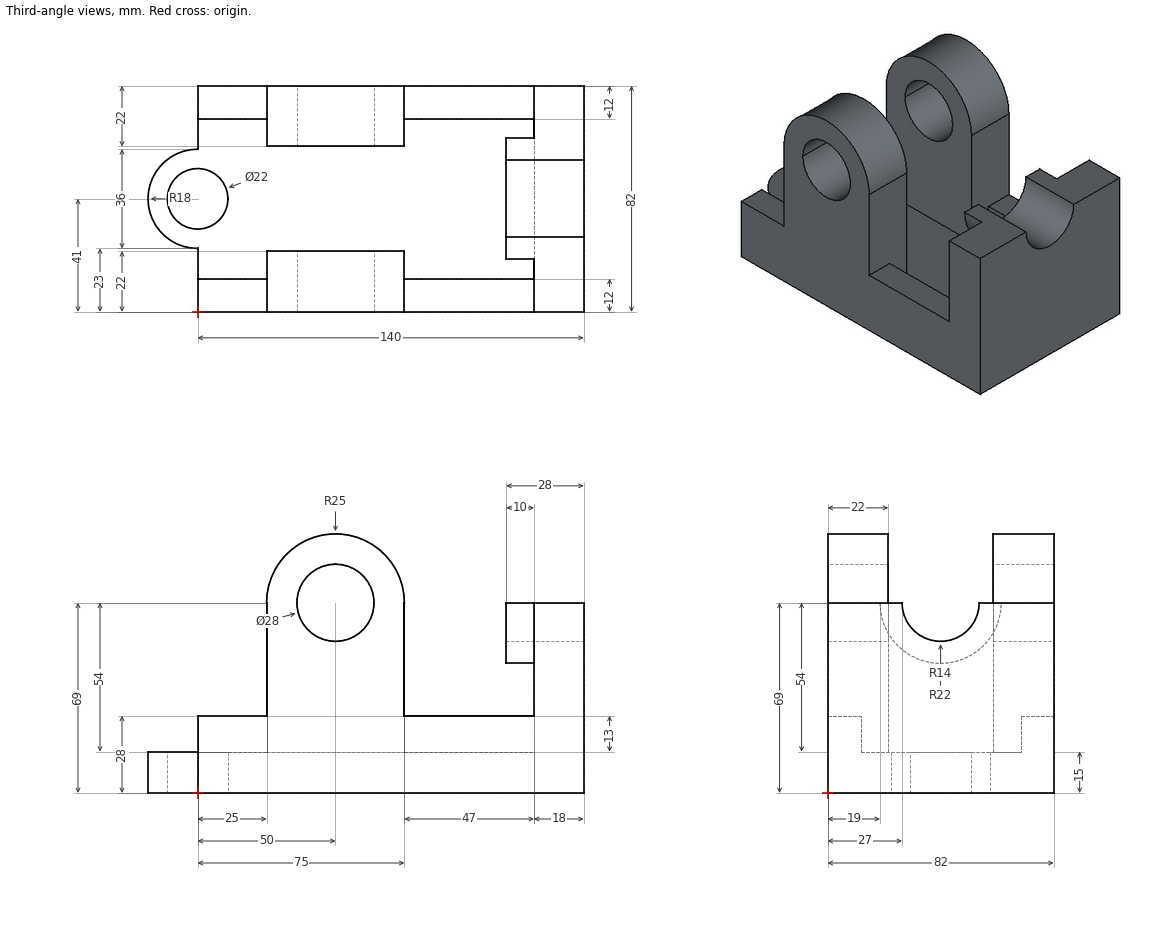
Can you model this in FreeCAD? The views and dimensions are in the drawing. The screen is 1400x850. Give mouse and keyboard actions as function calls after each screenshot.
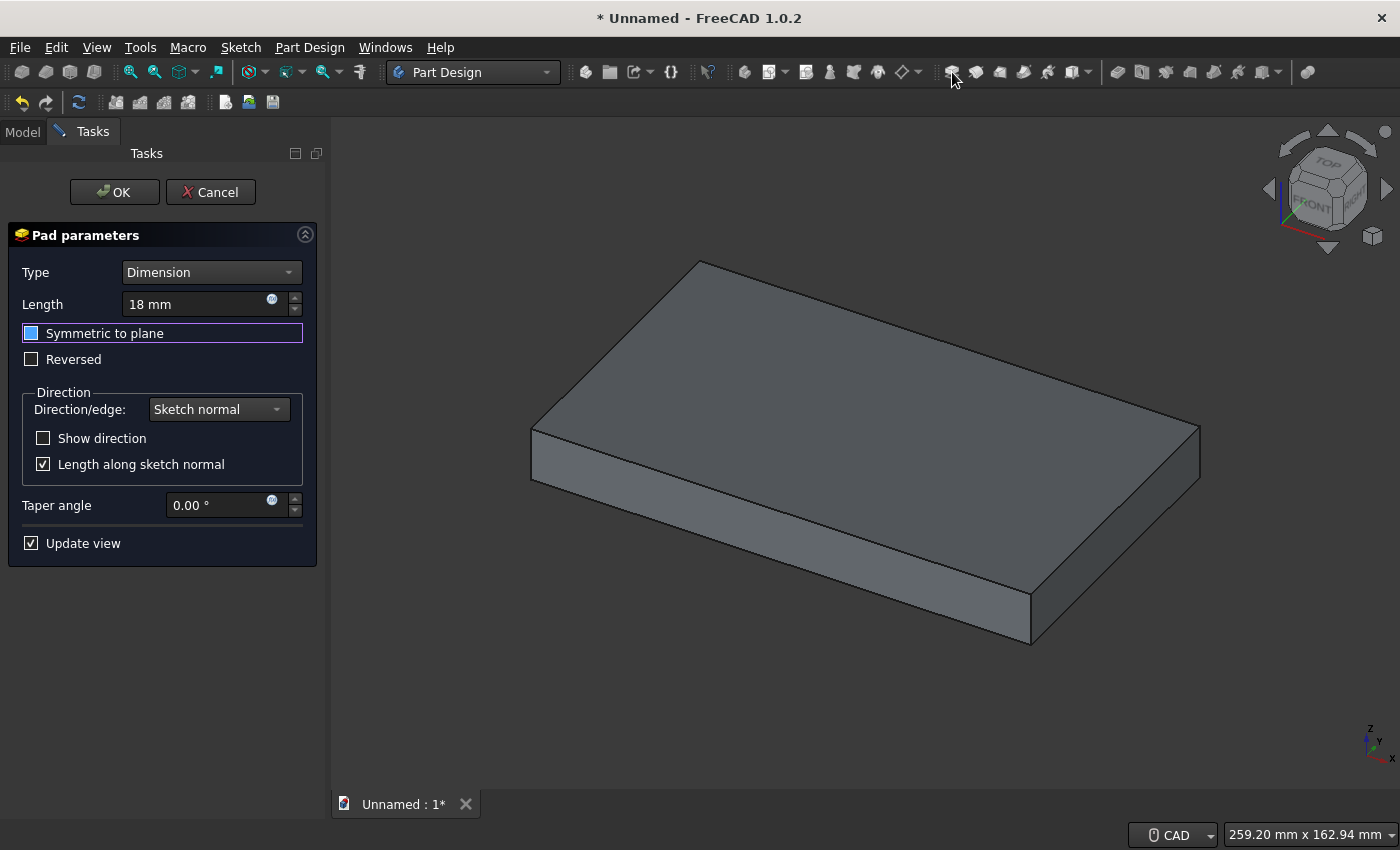
click(30, 359)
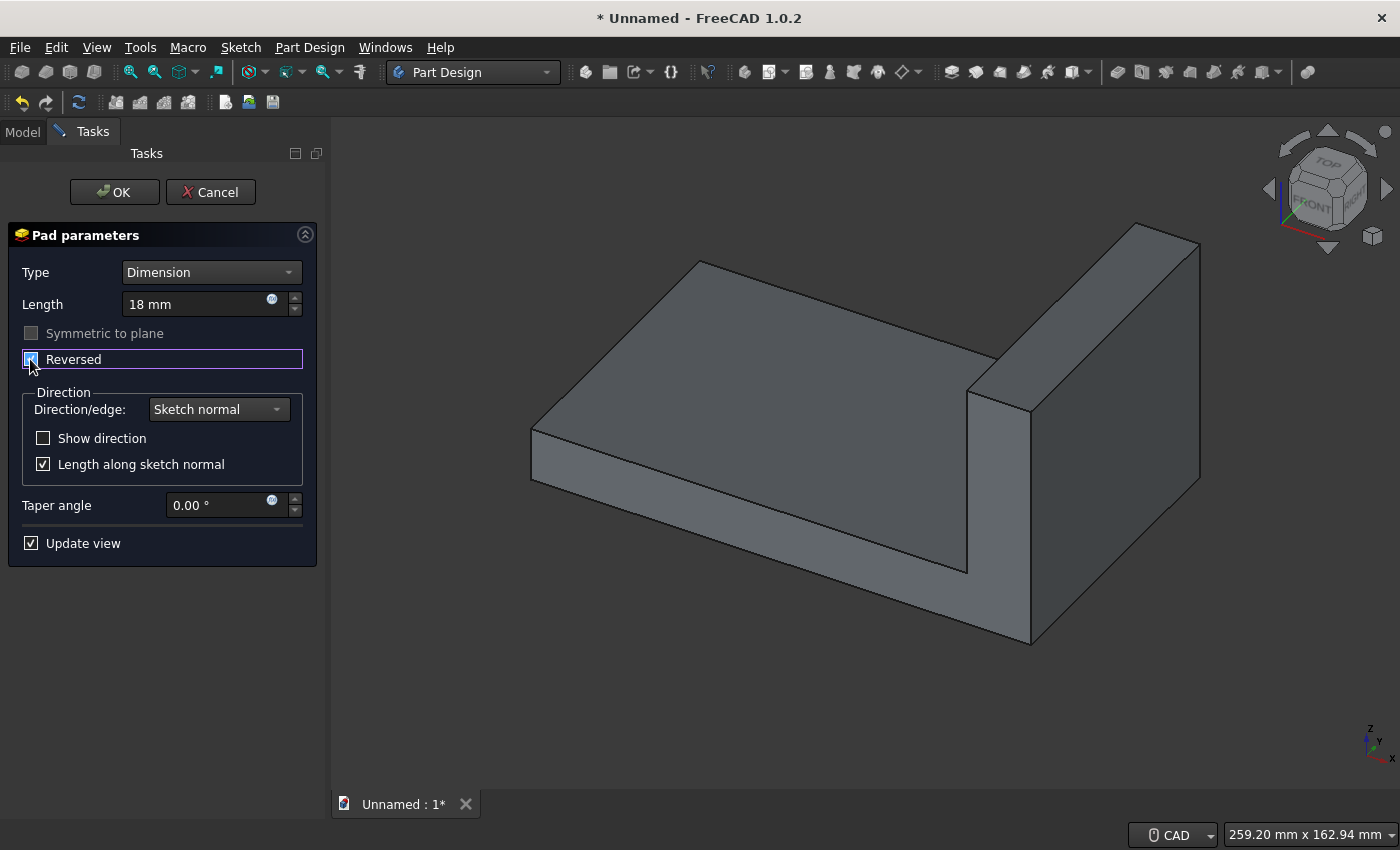
click(115, 192)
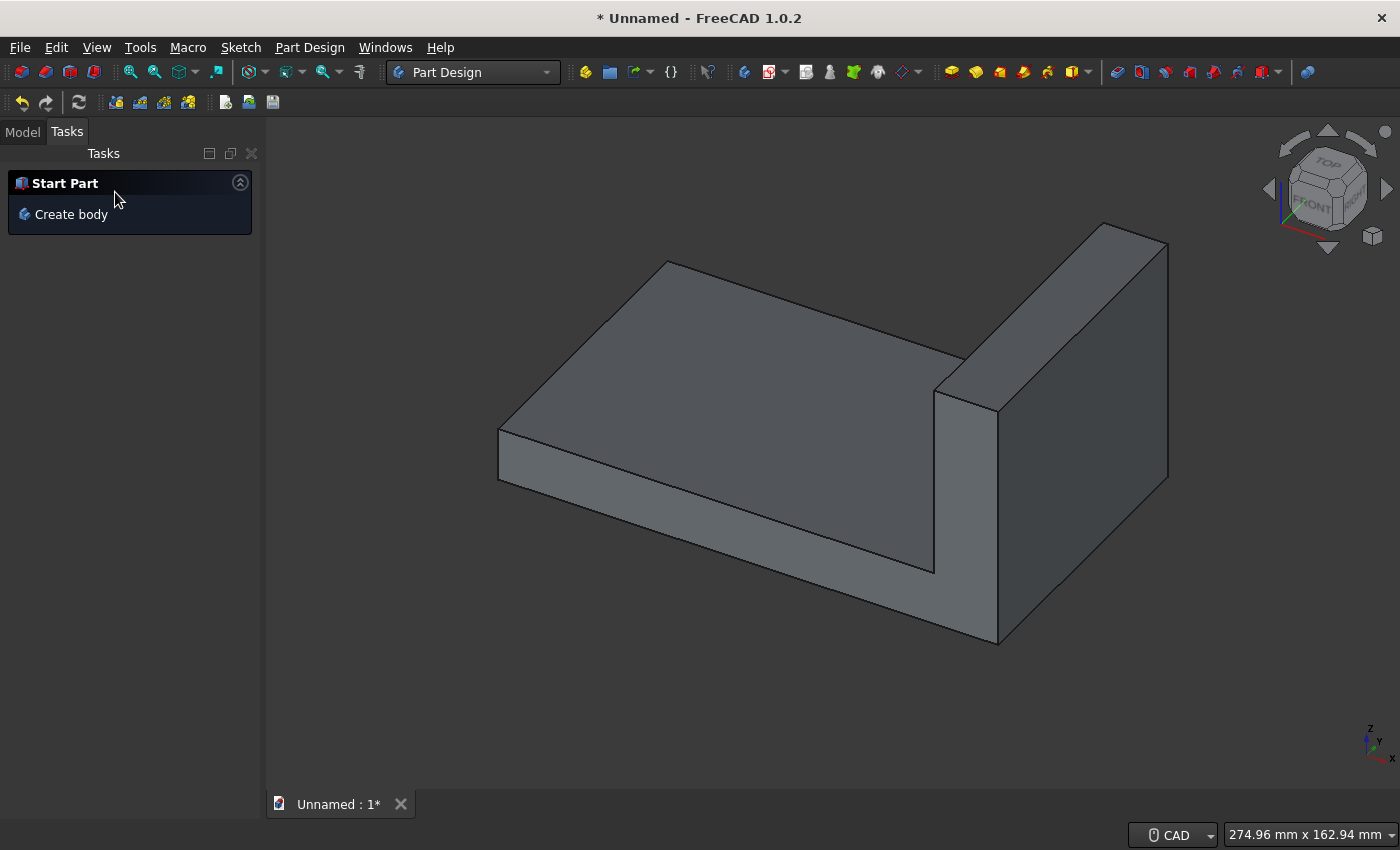
click(132, 72)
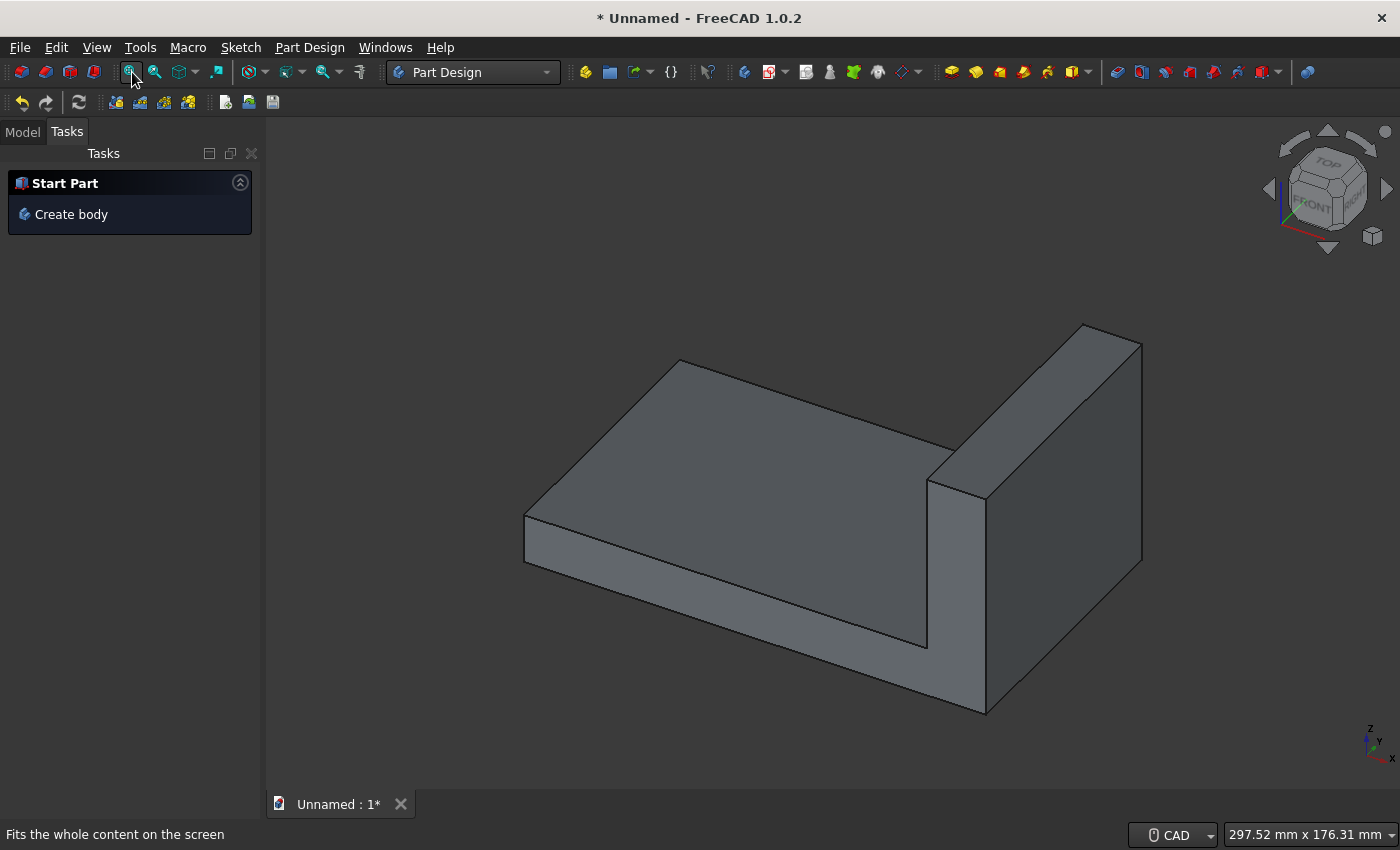
key(6)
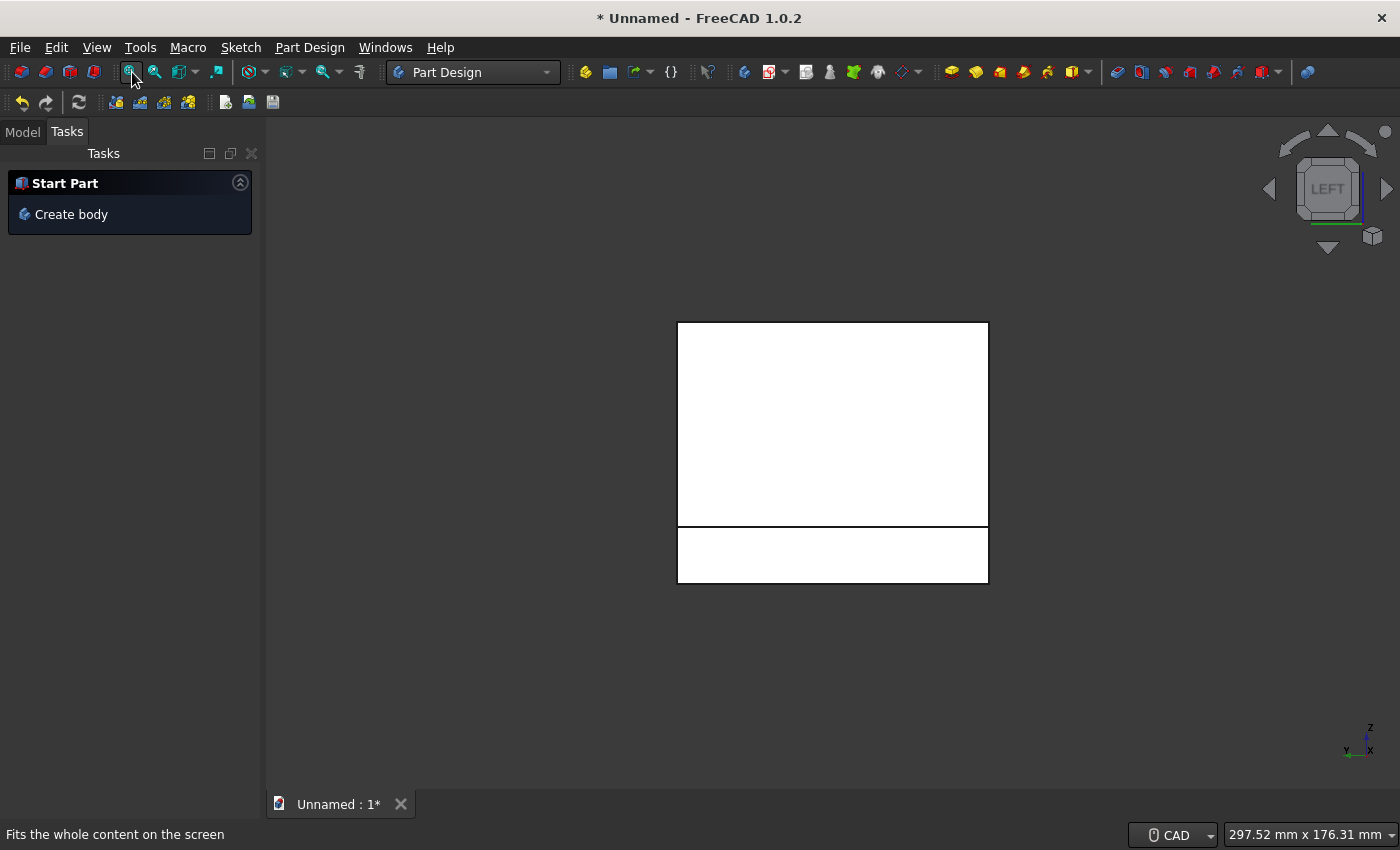
click(132, 72)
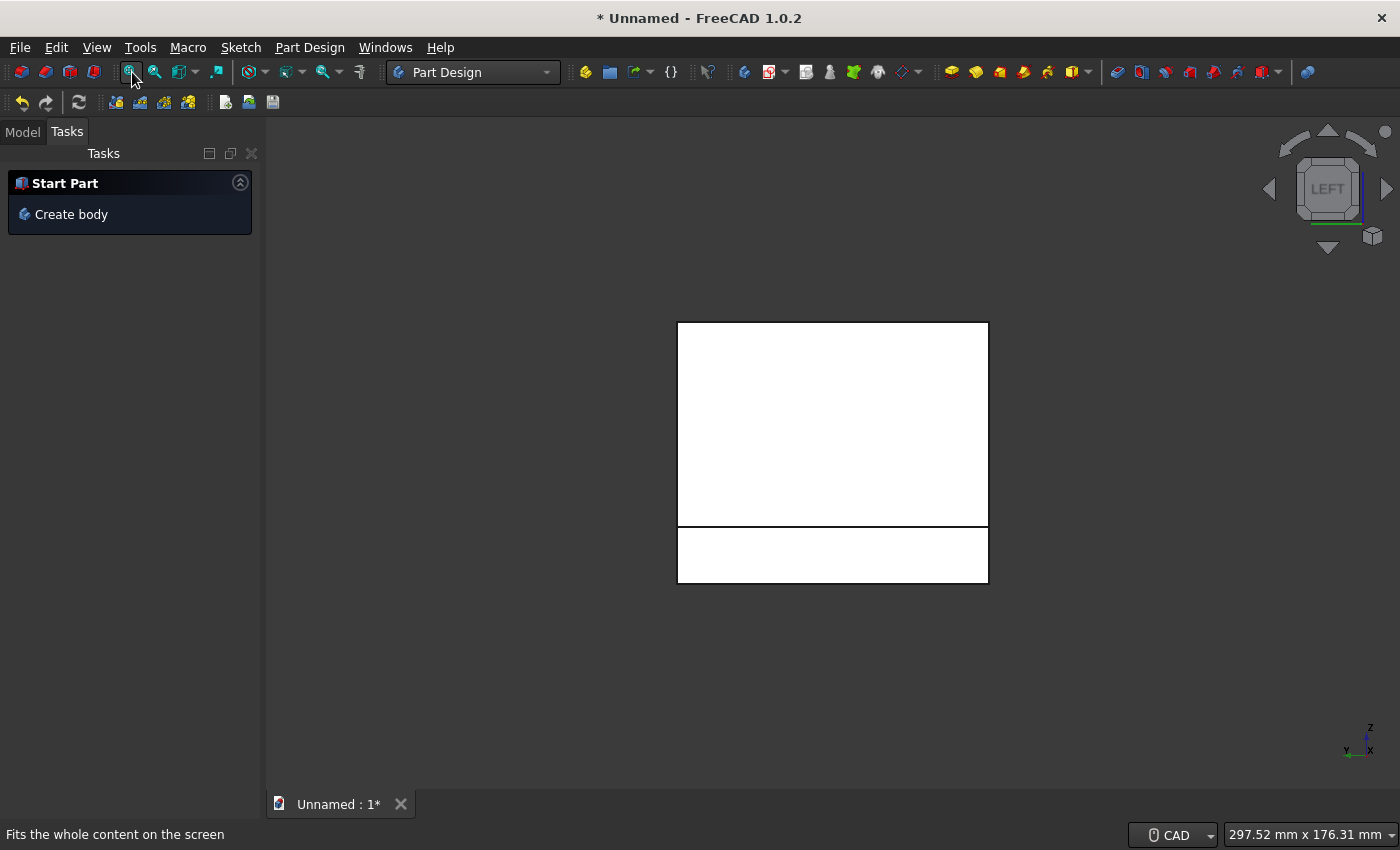
click(788, 423)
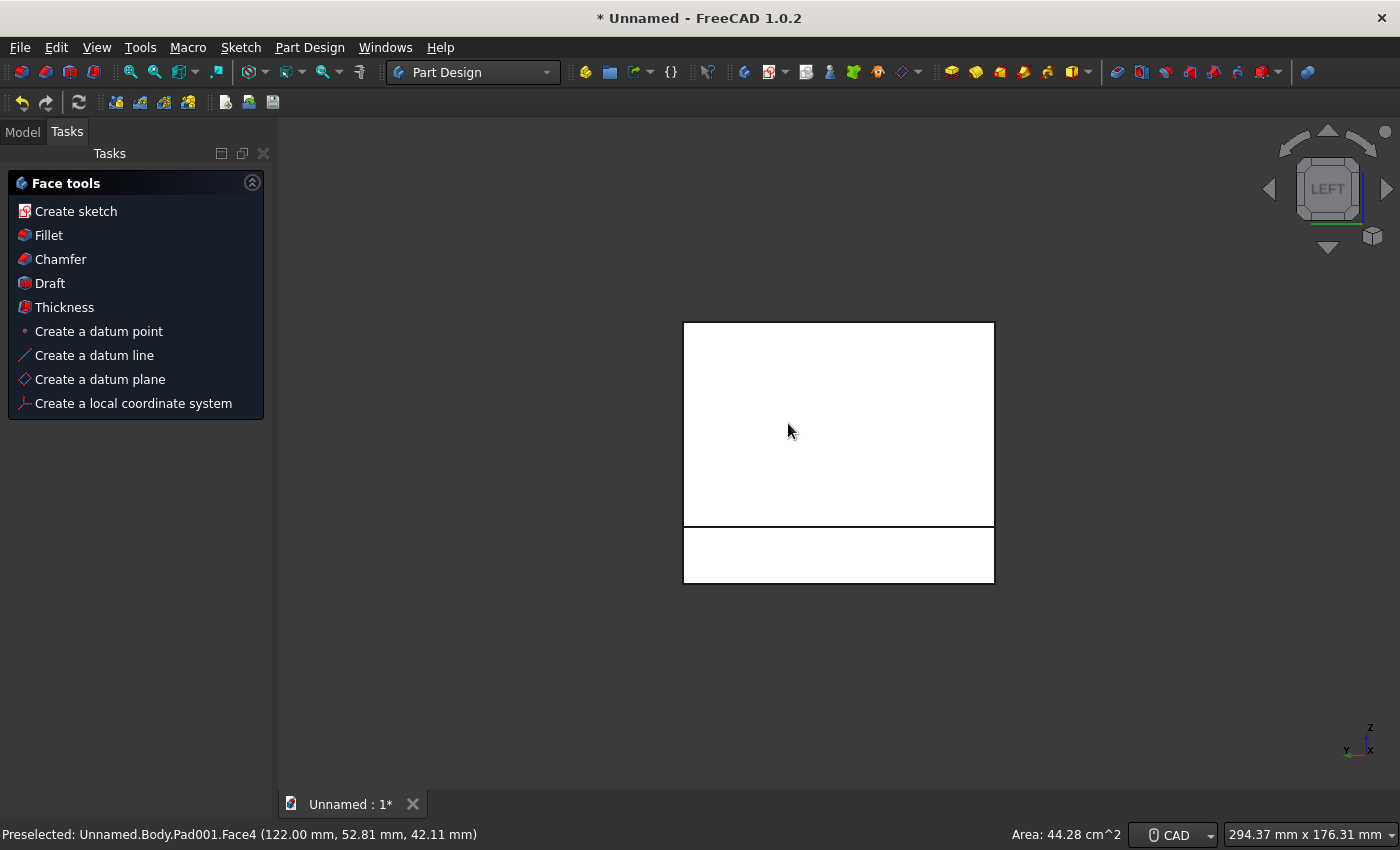
click(770, 72)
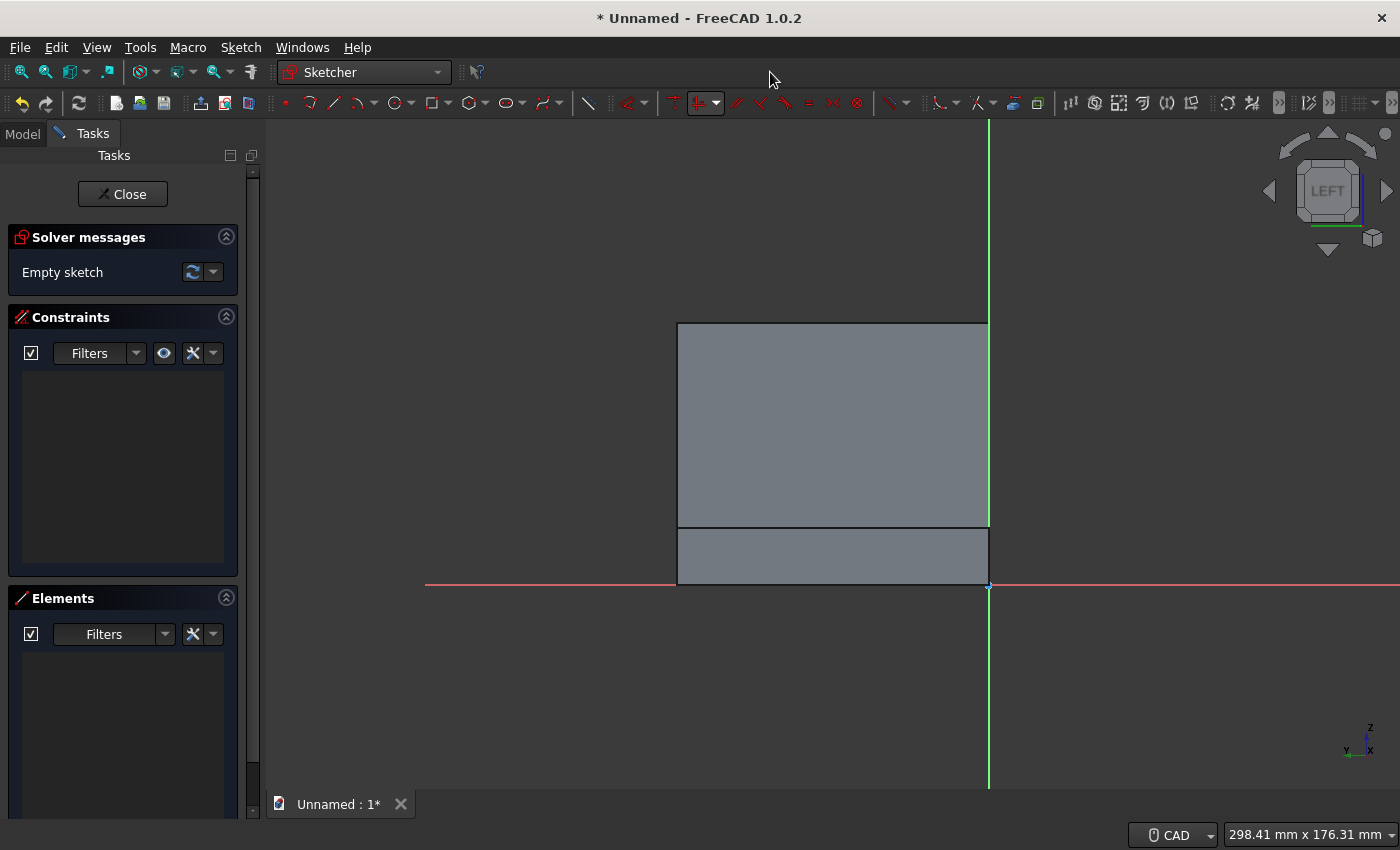
scroll(996, 454, up, 3)